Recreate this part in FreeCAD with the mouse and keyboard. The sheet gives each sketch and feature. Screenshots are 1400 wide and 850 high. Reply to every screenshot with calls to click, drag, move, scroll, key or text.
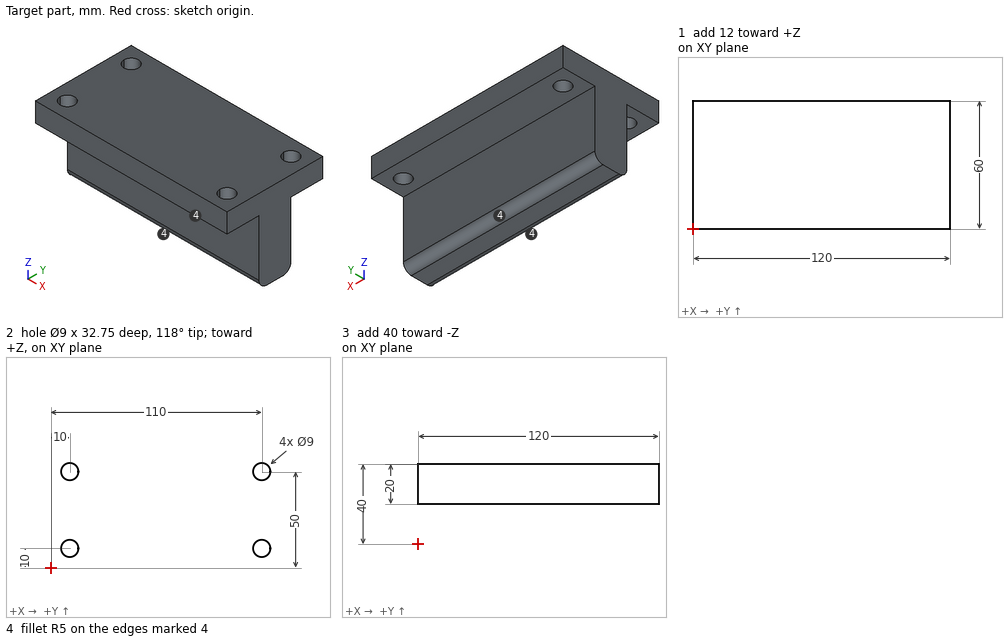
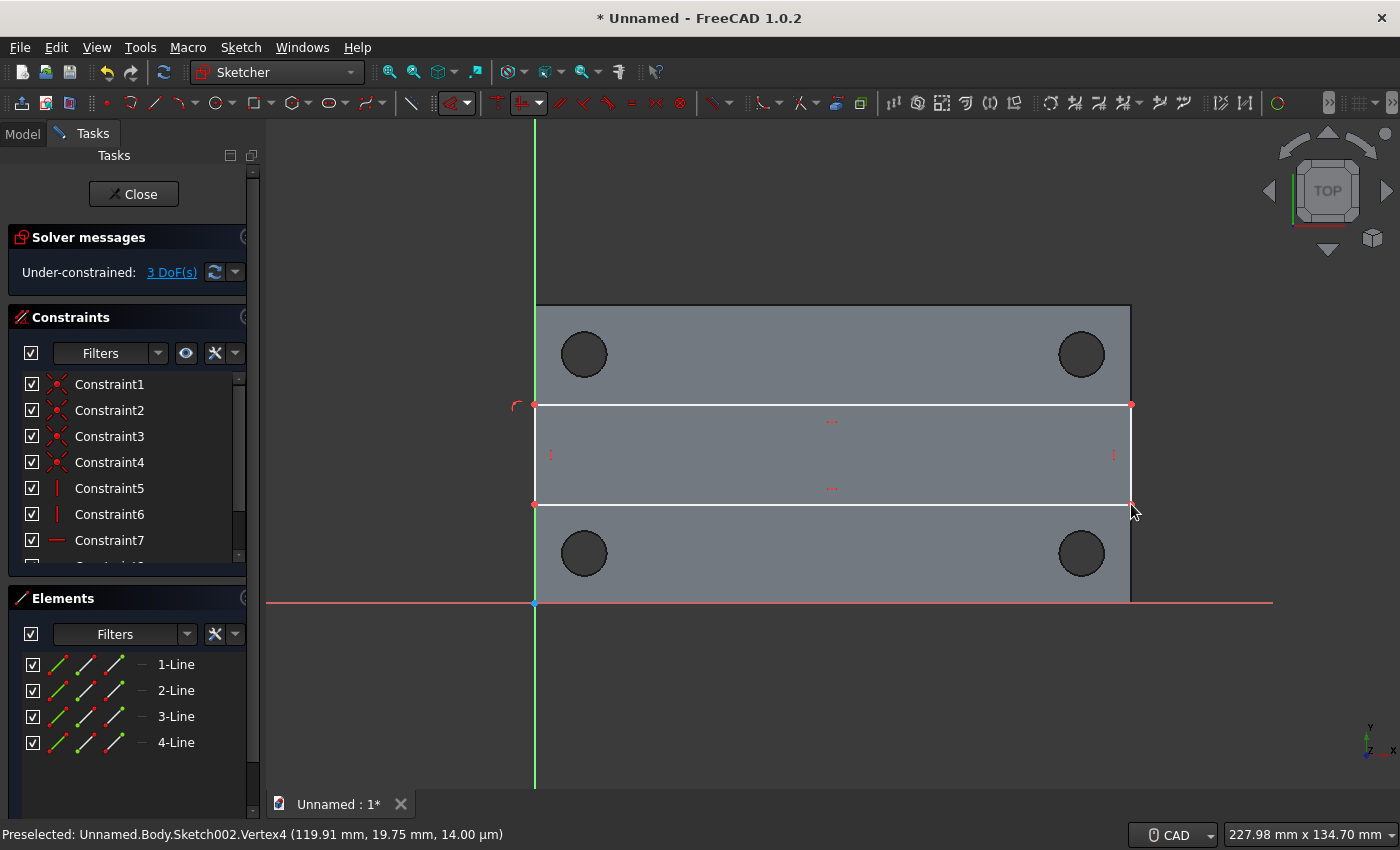
click(535, 435)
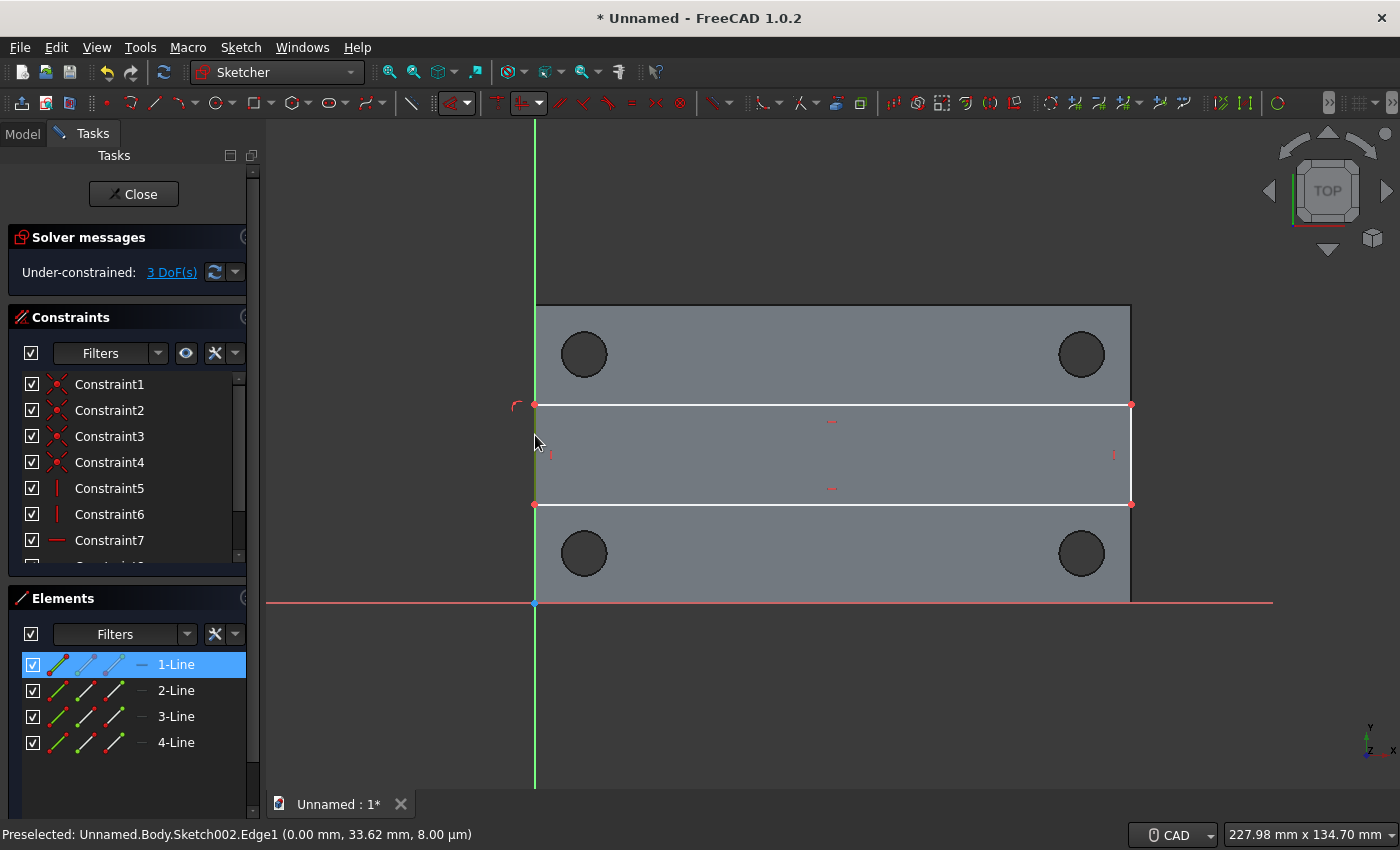
key(i)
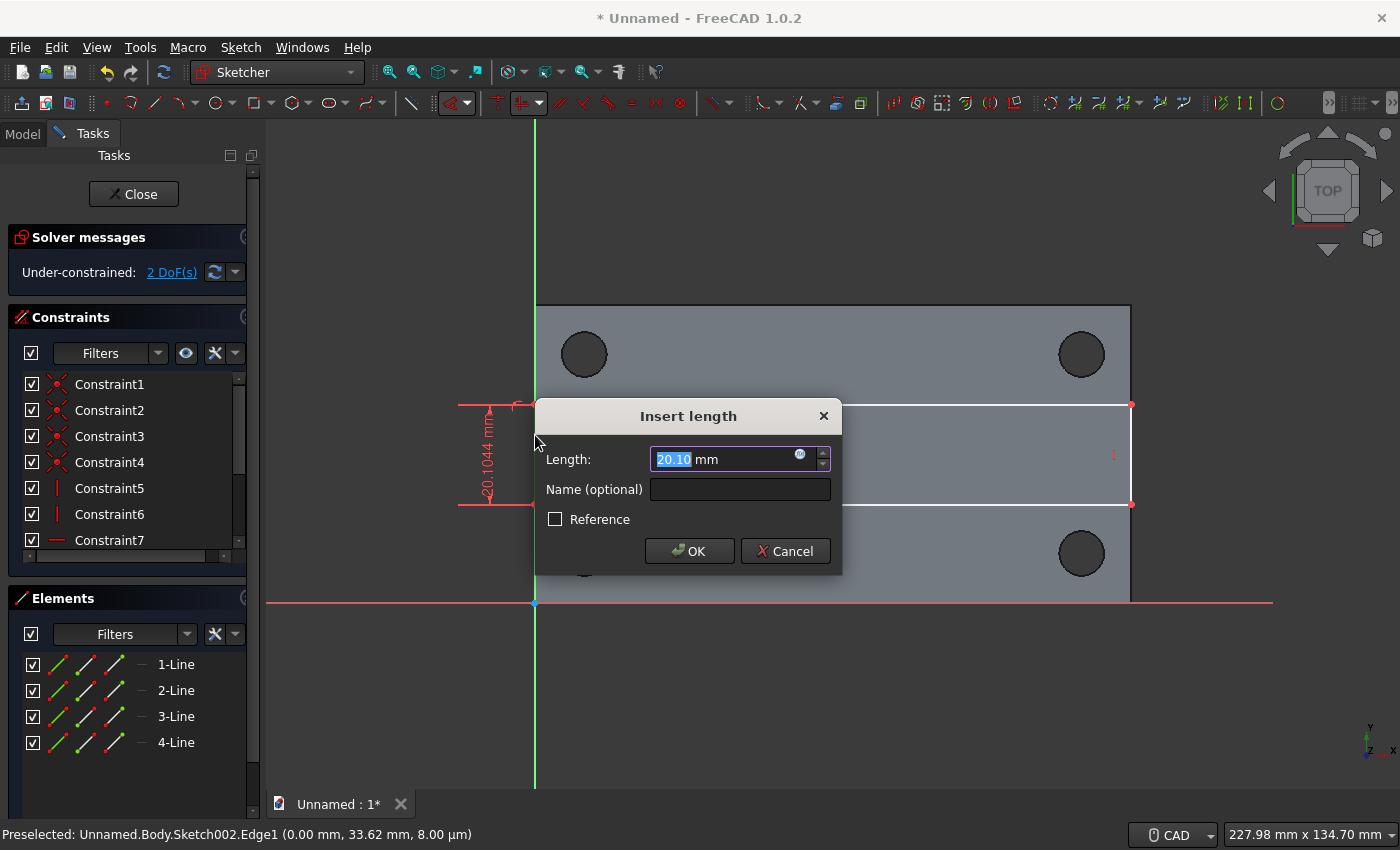
text(20)
key(Return)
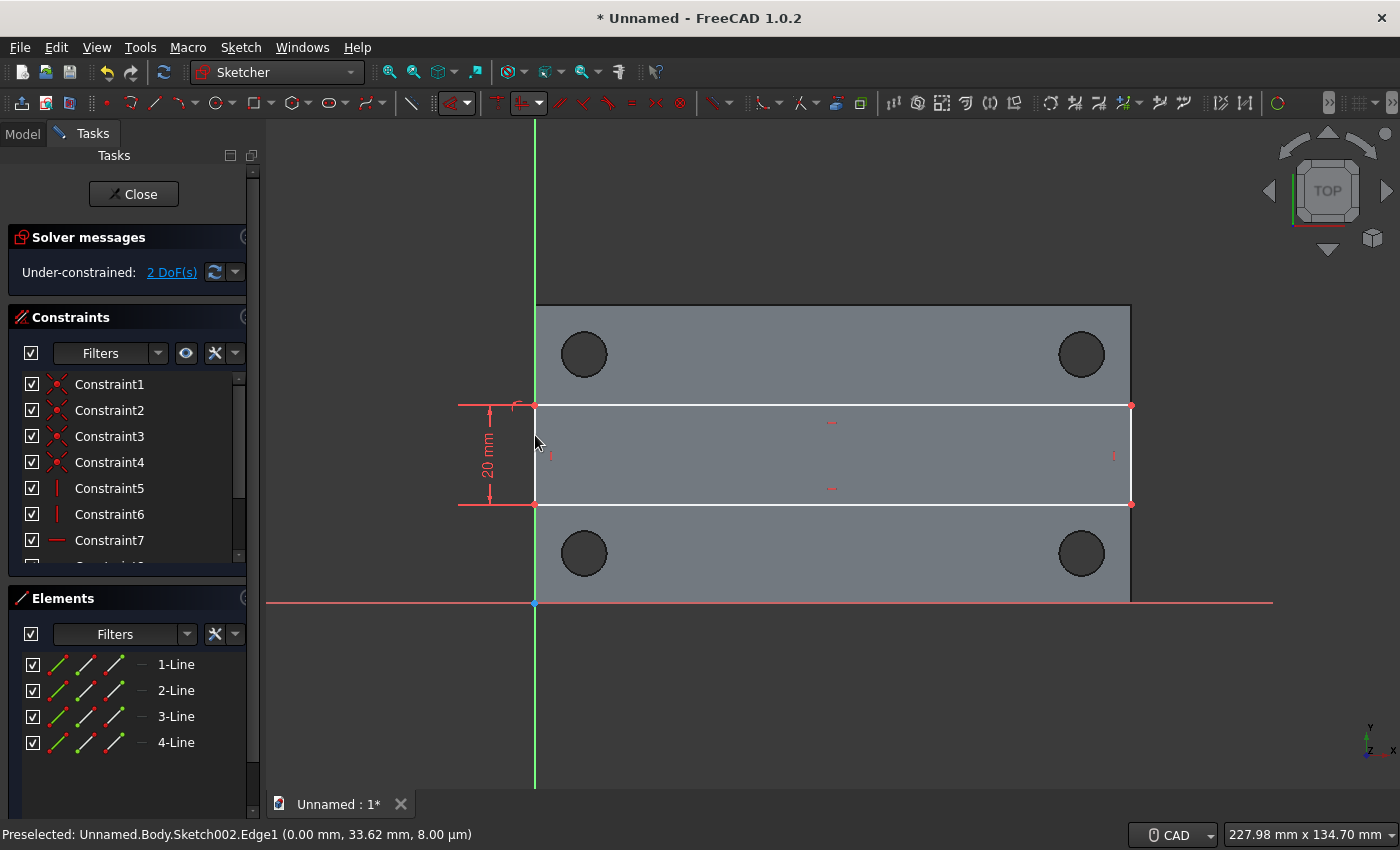
click(713, 505)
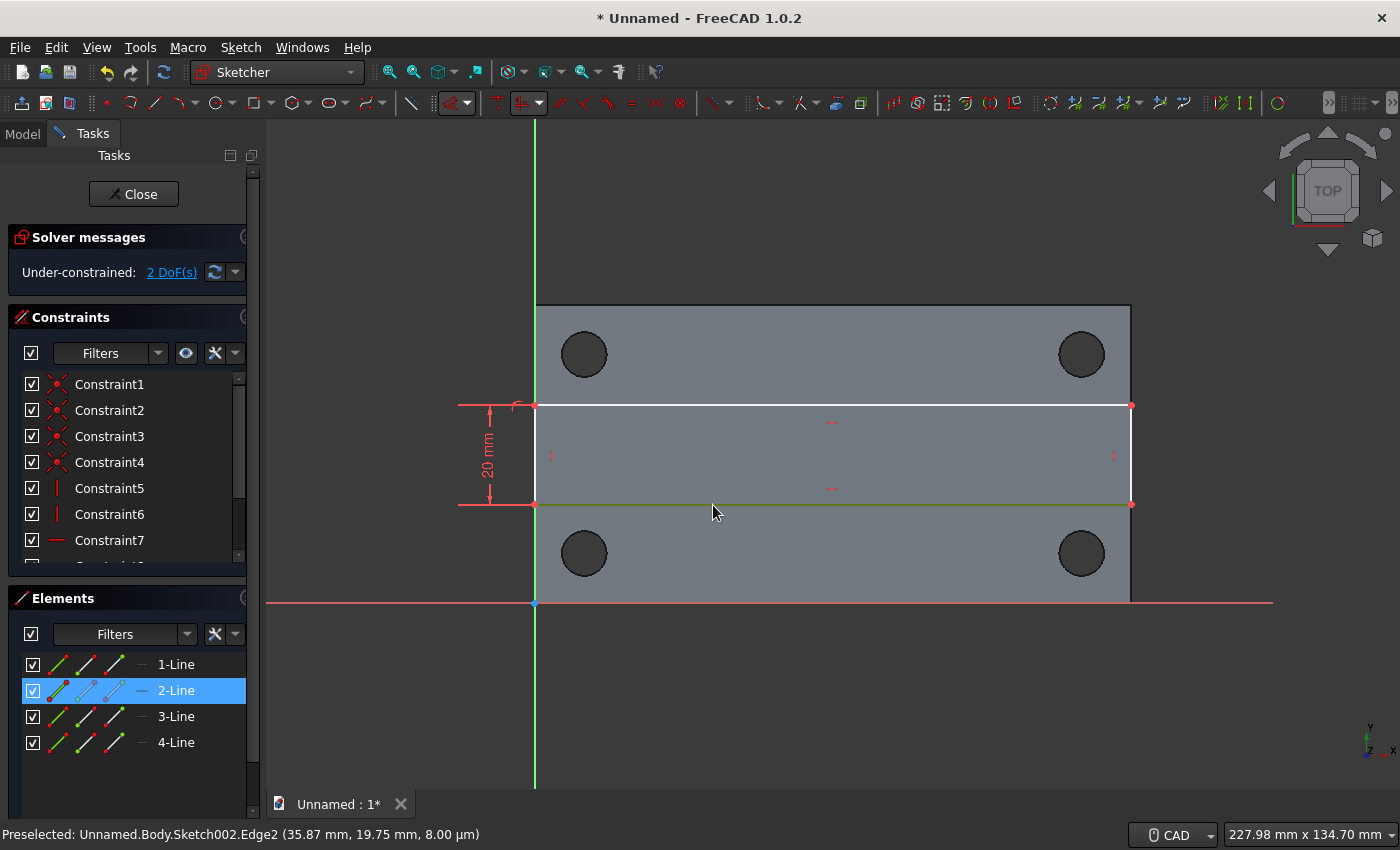
click(470, 104)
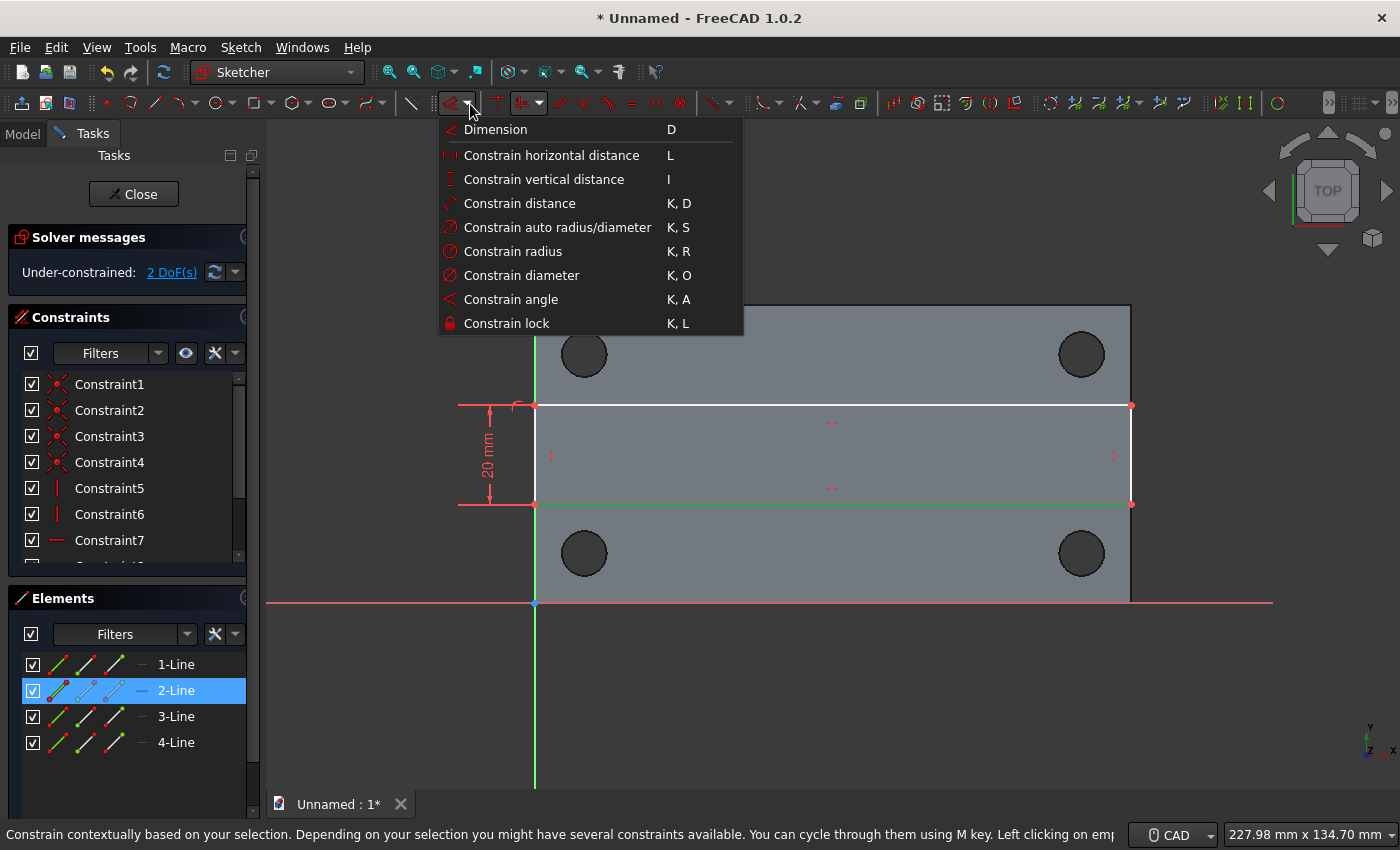
click(591, 155)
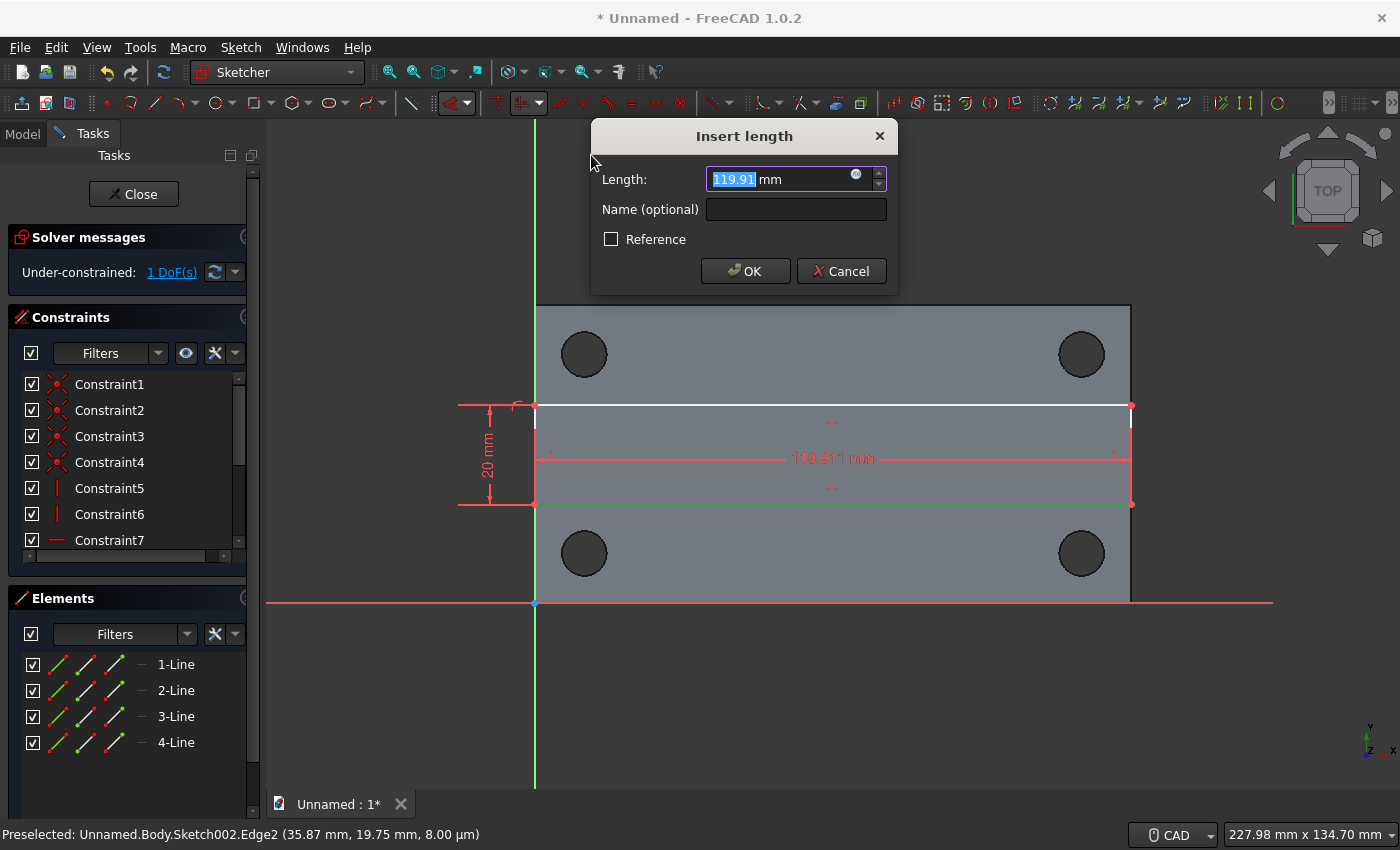
text(120)
key(Return)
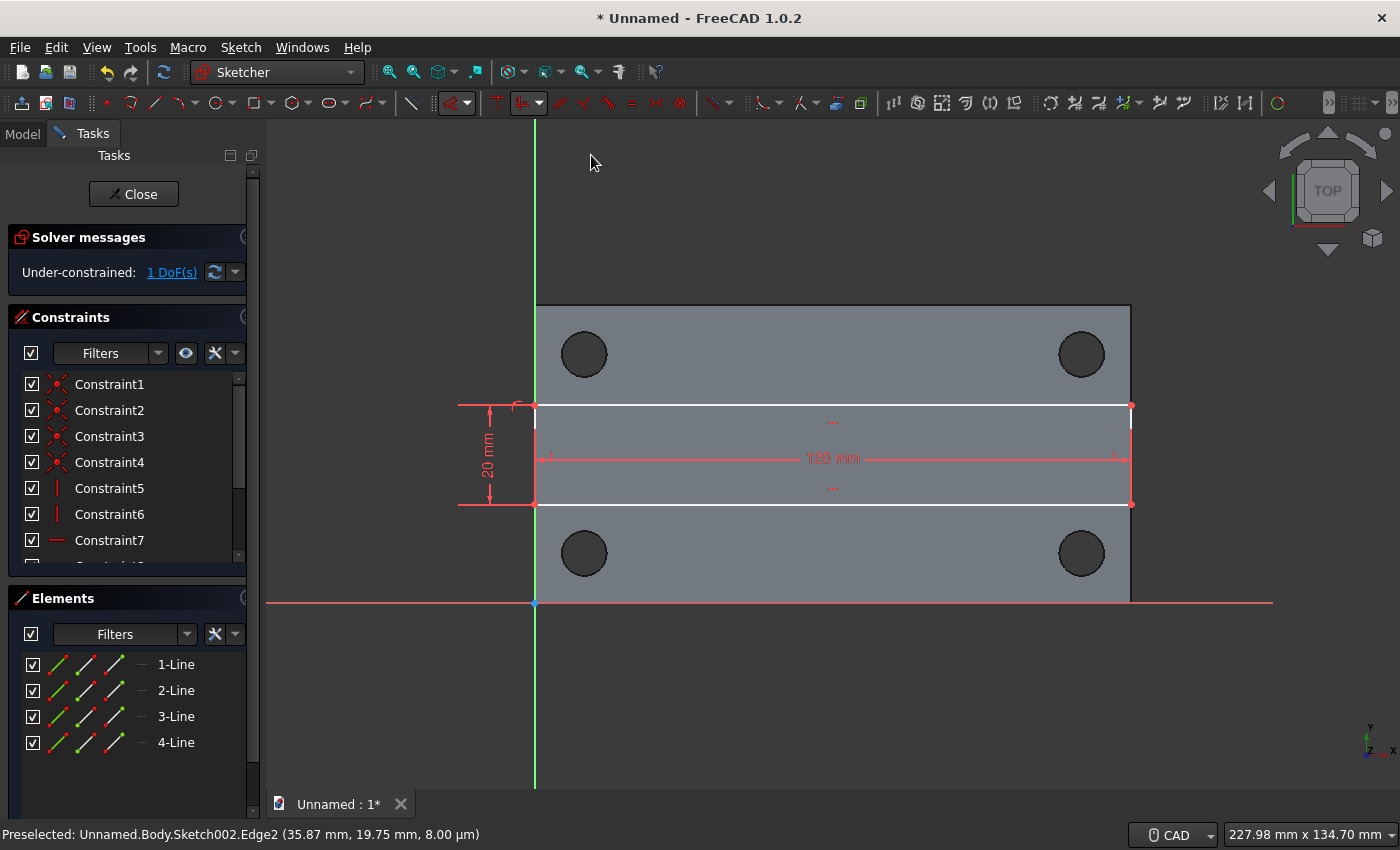
click(535, 405)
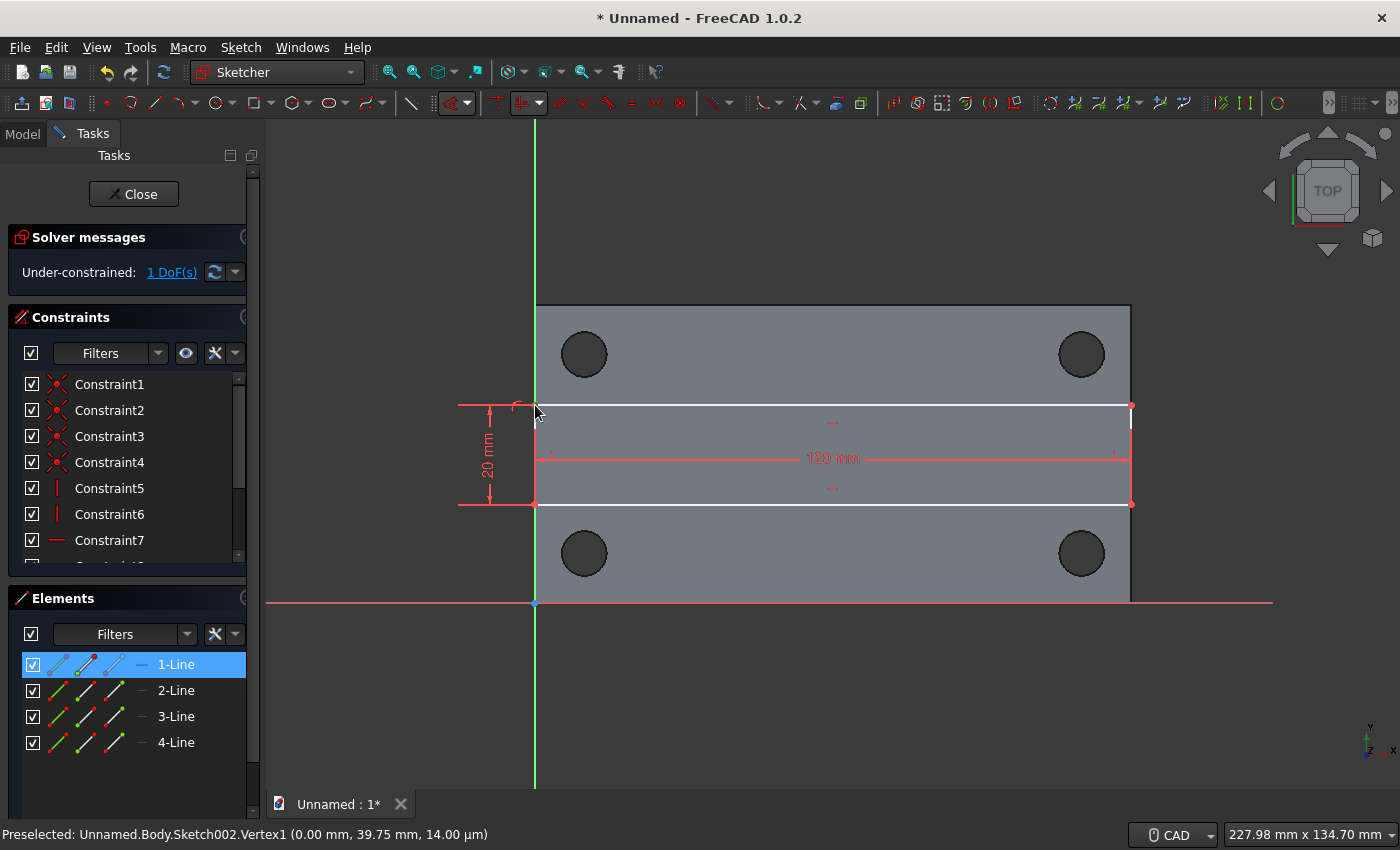
click(470, 104)